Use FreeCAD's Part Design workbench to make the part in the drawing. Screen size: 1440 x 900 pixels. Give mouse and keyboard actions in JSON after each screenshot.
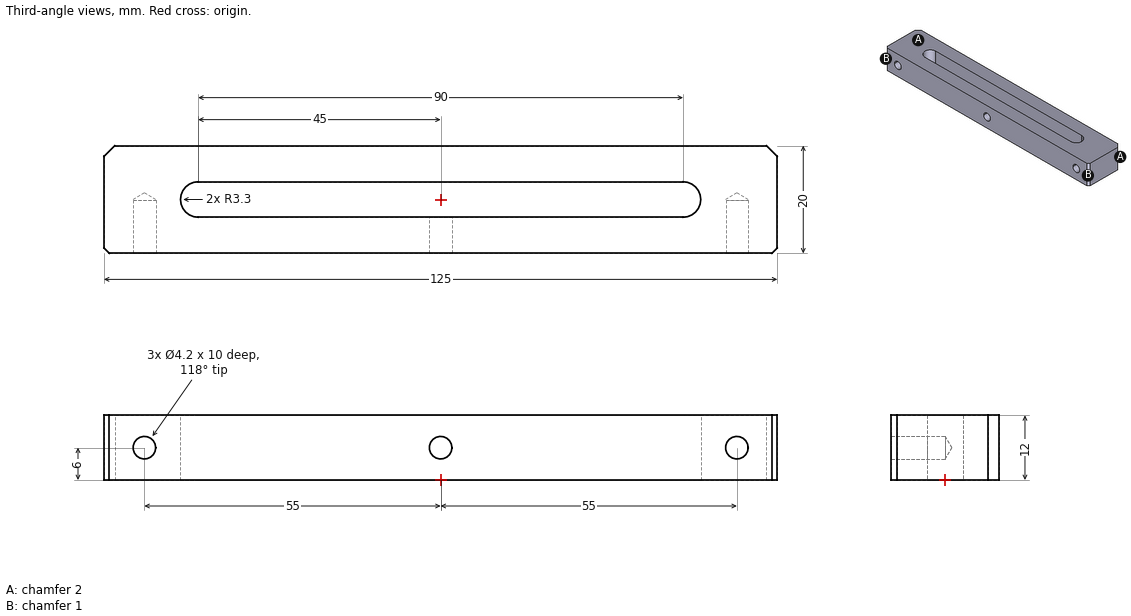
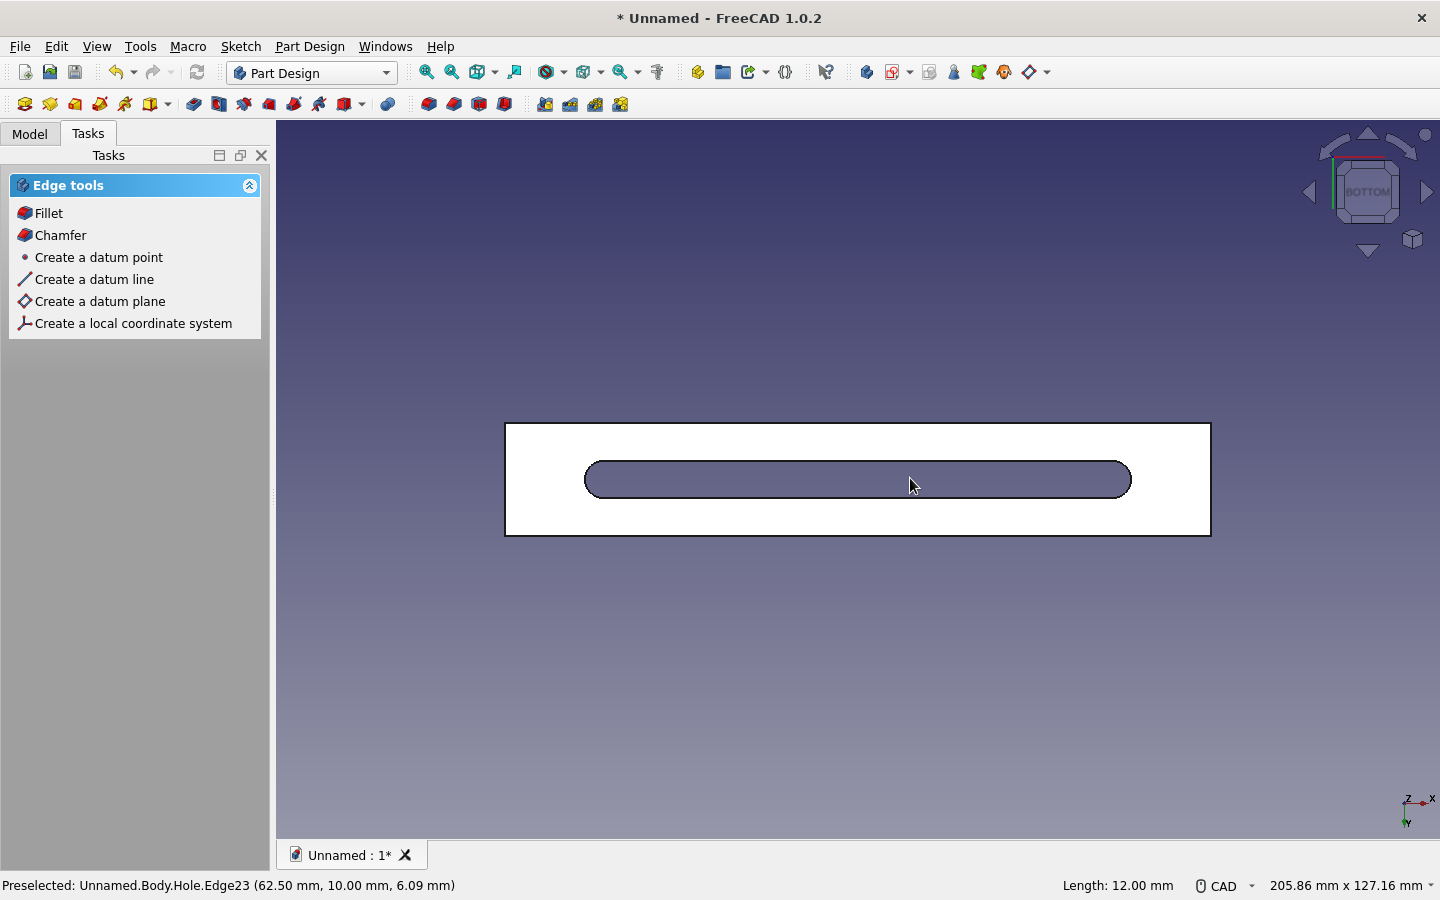
{"action": "key", "text": "4"}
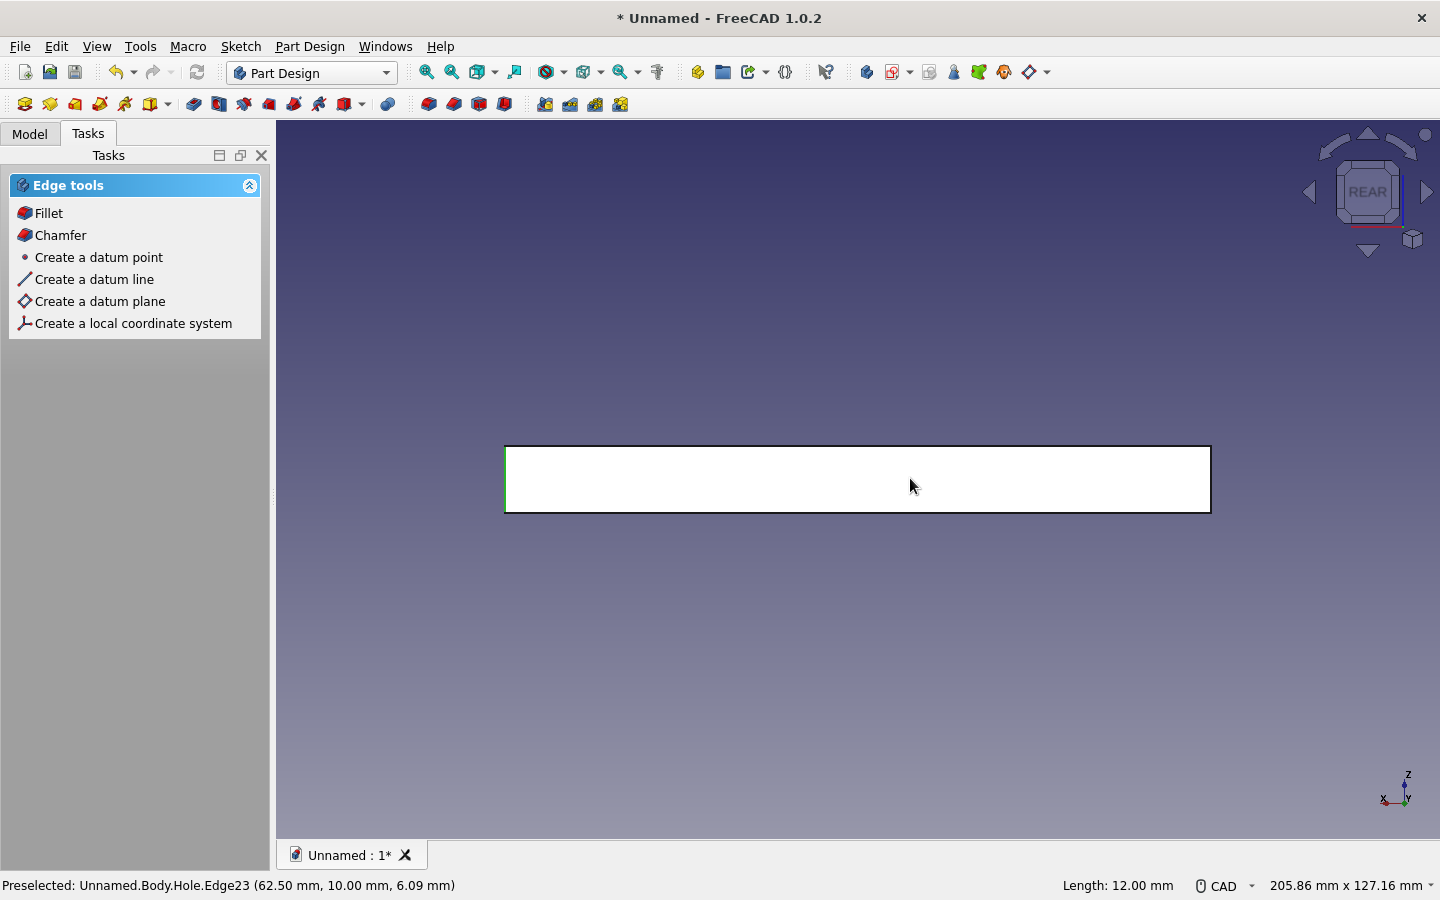
{"action": "left_click", "coordinate": [1211, 479], "text": "ctrl"}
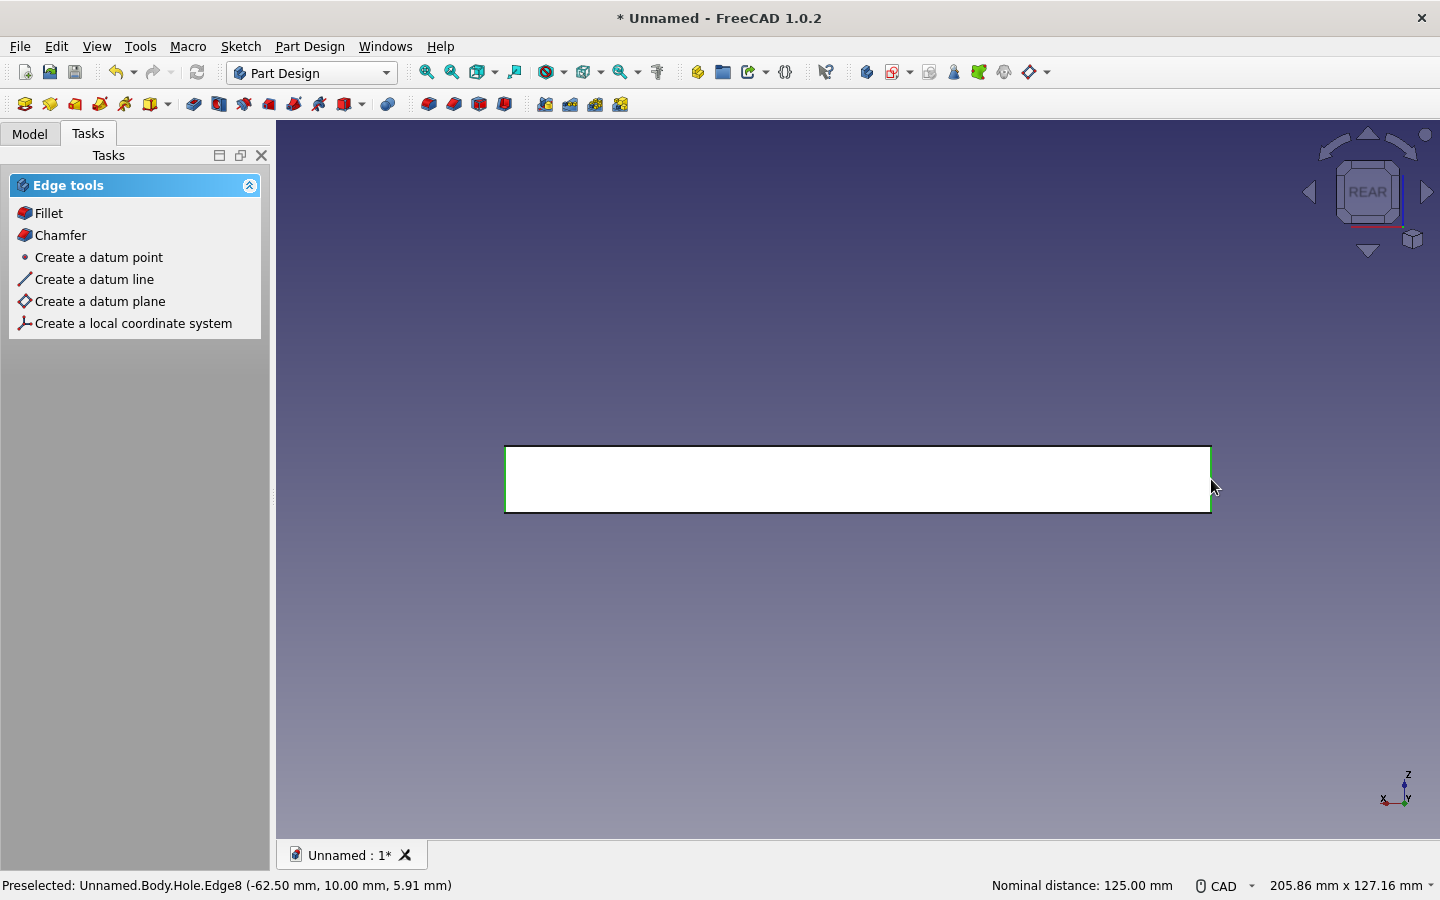
{"action": "left_click", "coordinate": [454, 104]}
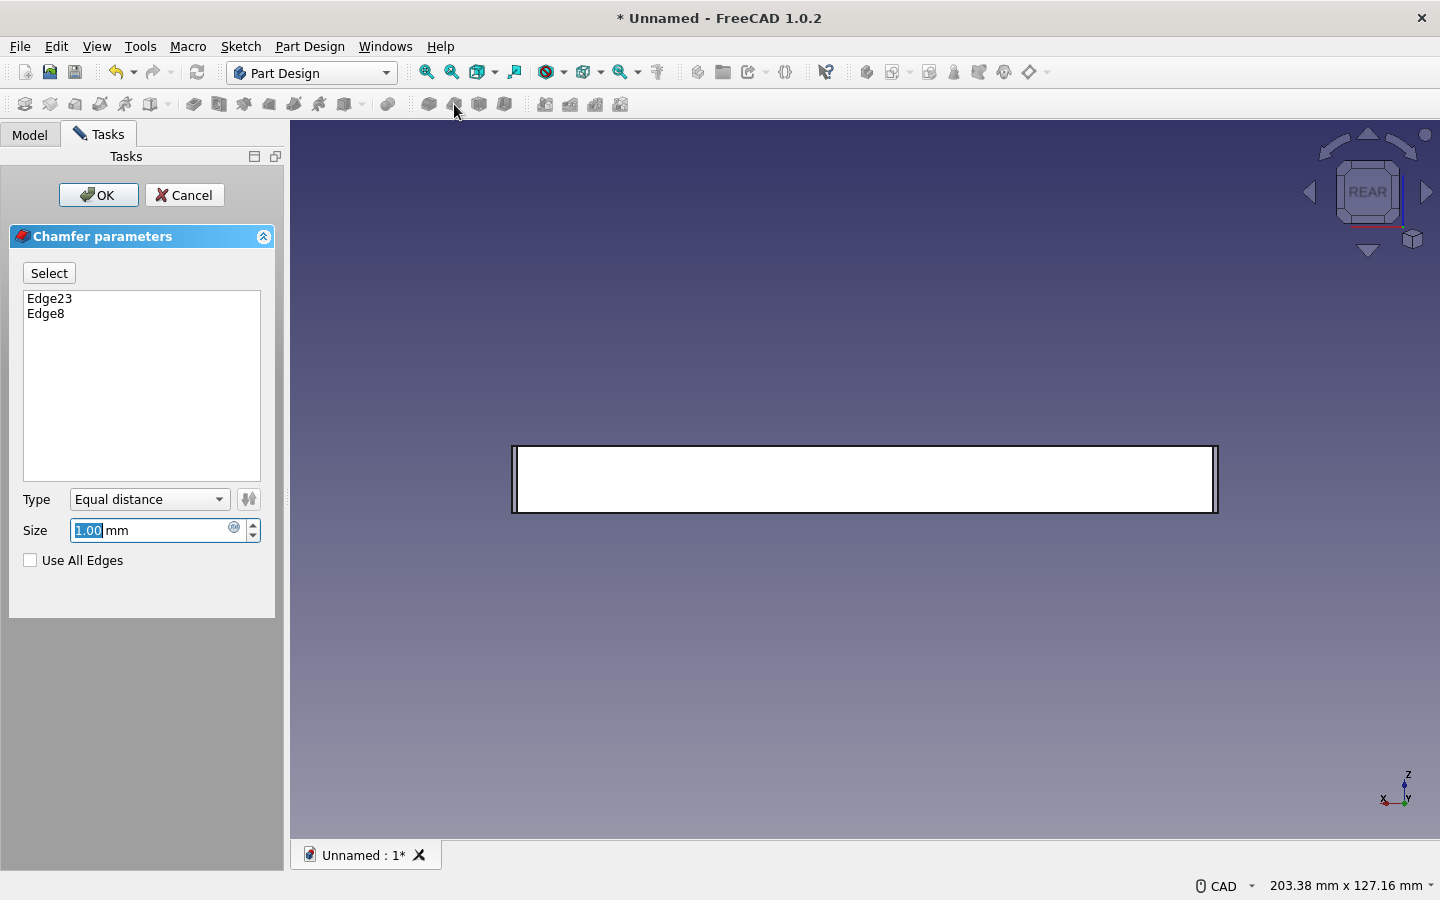
{"action": "type", "text": "2"}
{"action": "key", "text": "Tab"}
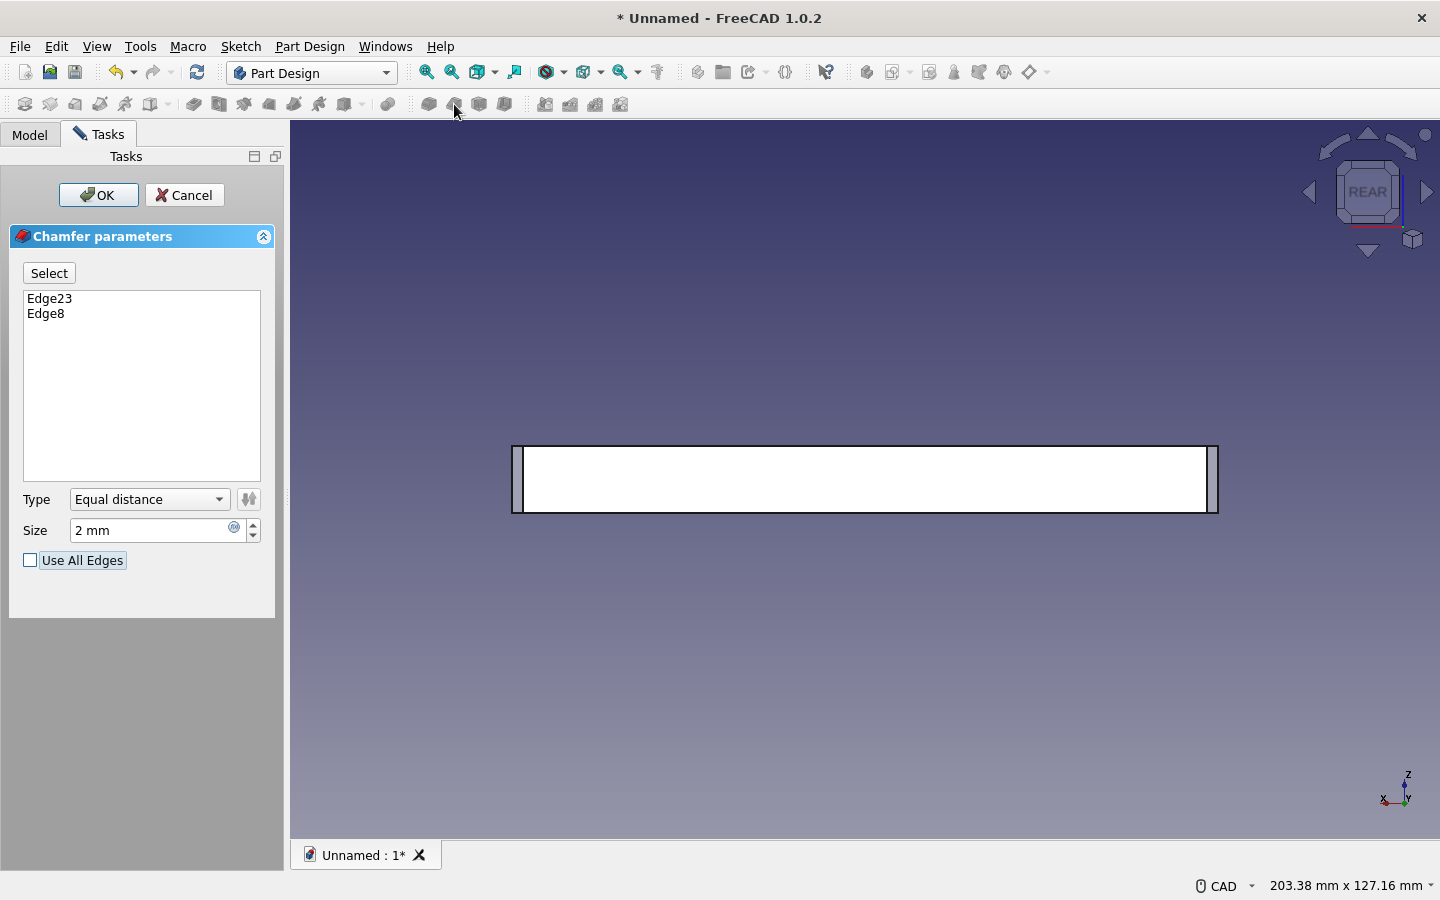
{"action": "left_click", "coordinate": [99, 195]}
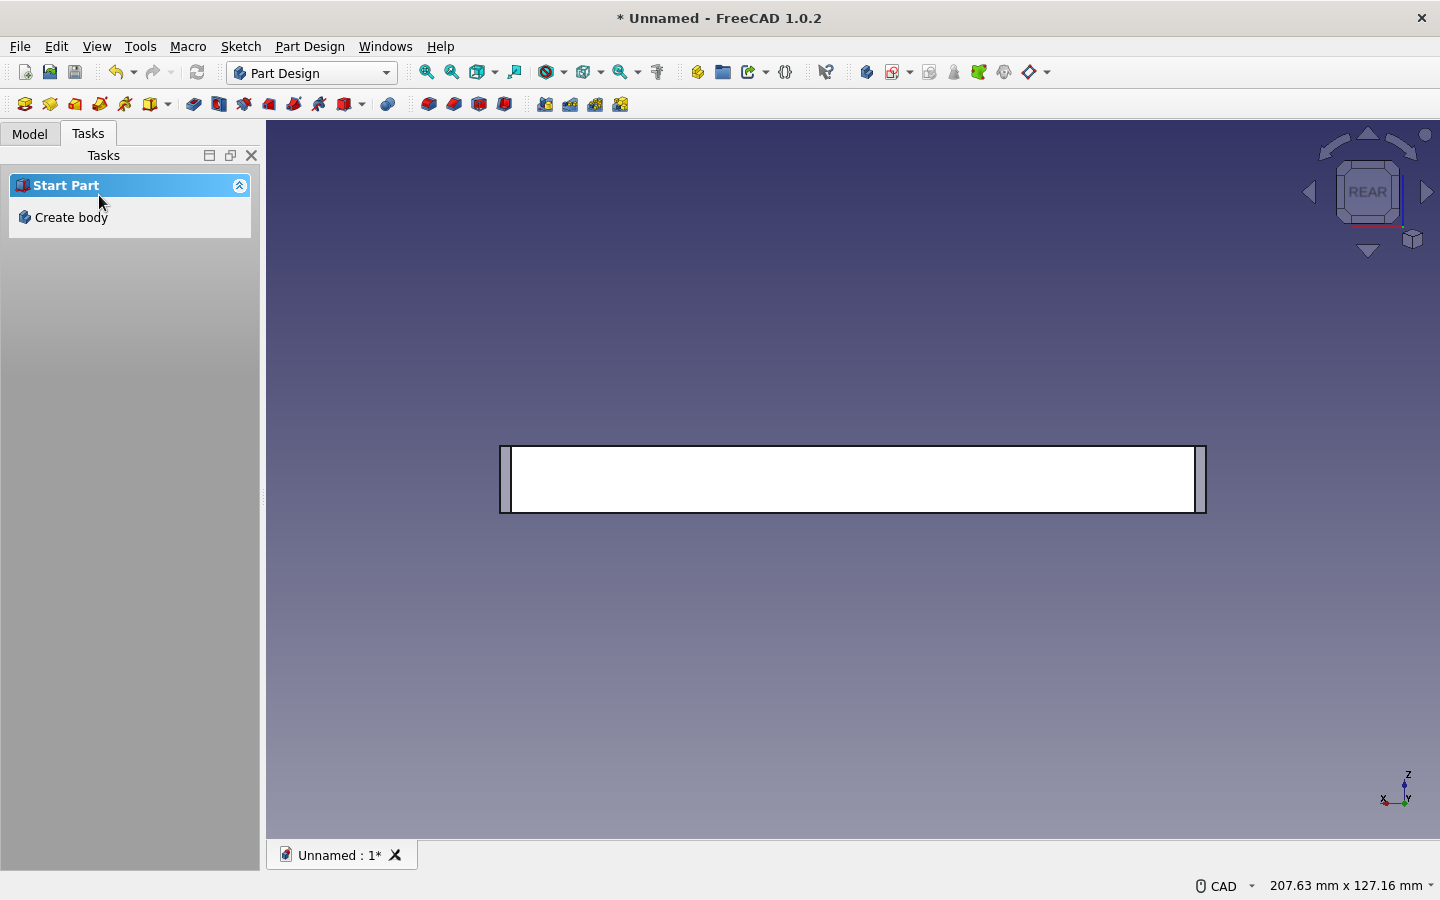
{"action": "key", "text": "0"}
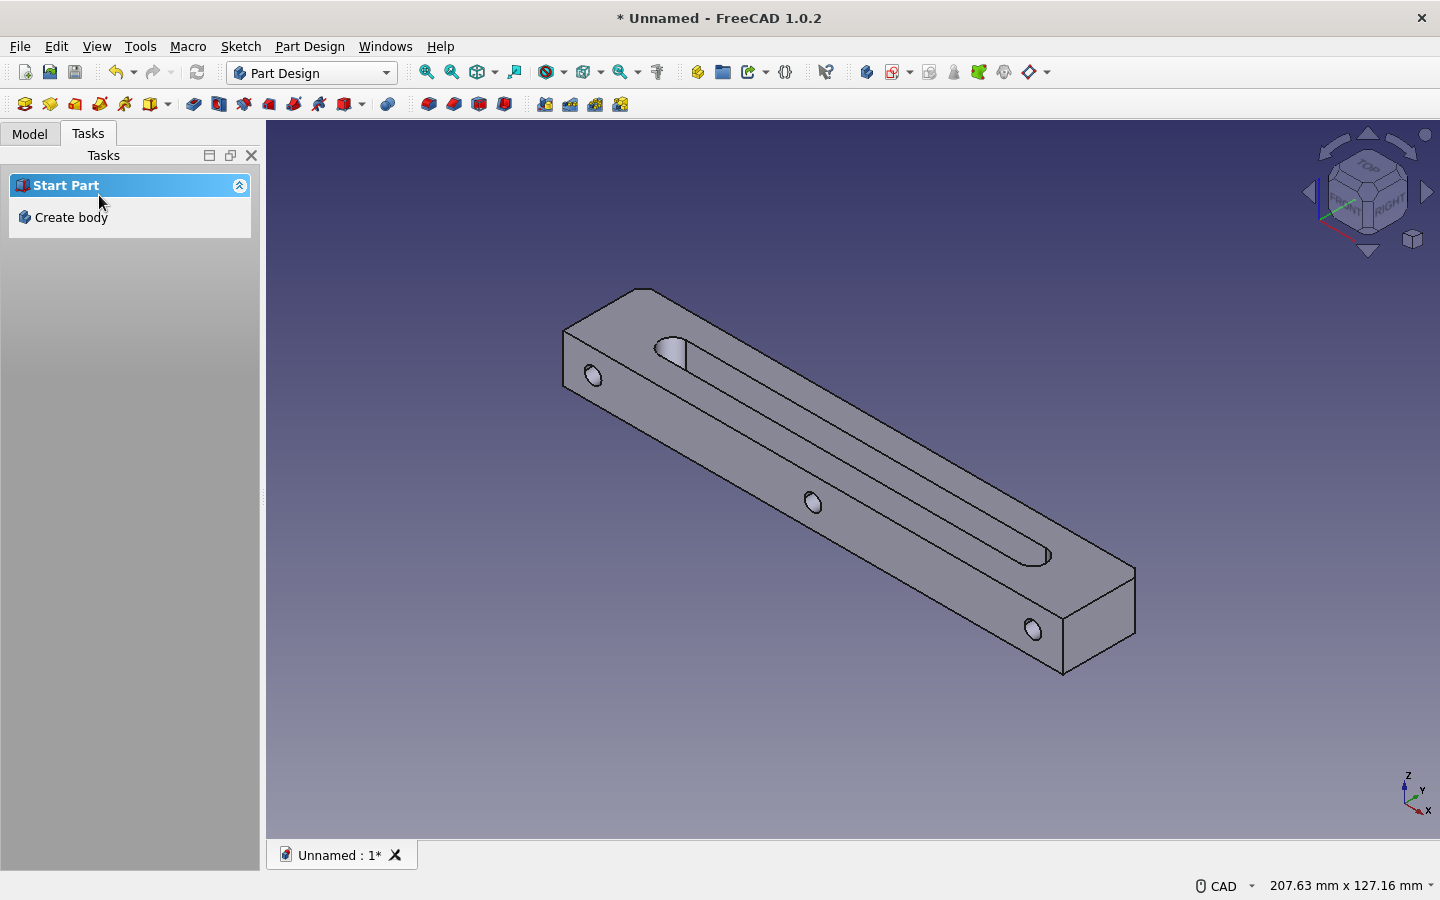
{"action": "left_click", "coordinate": [1063, 646]}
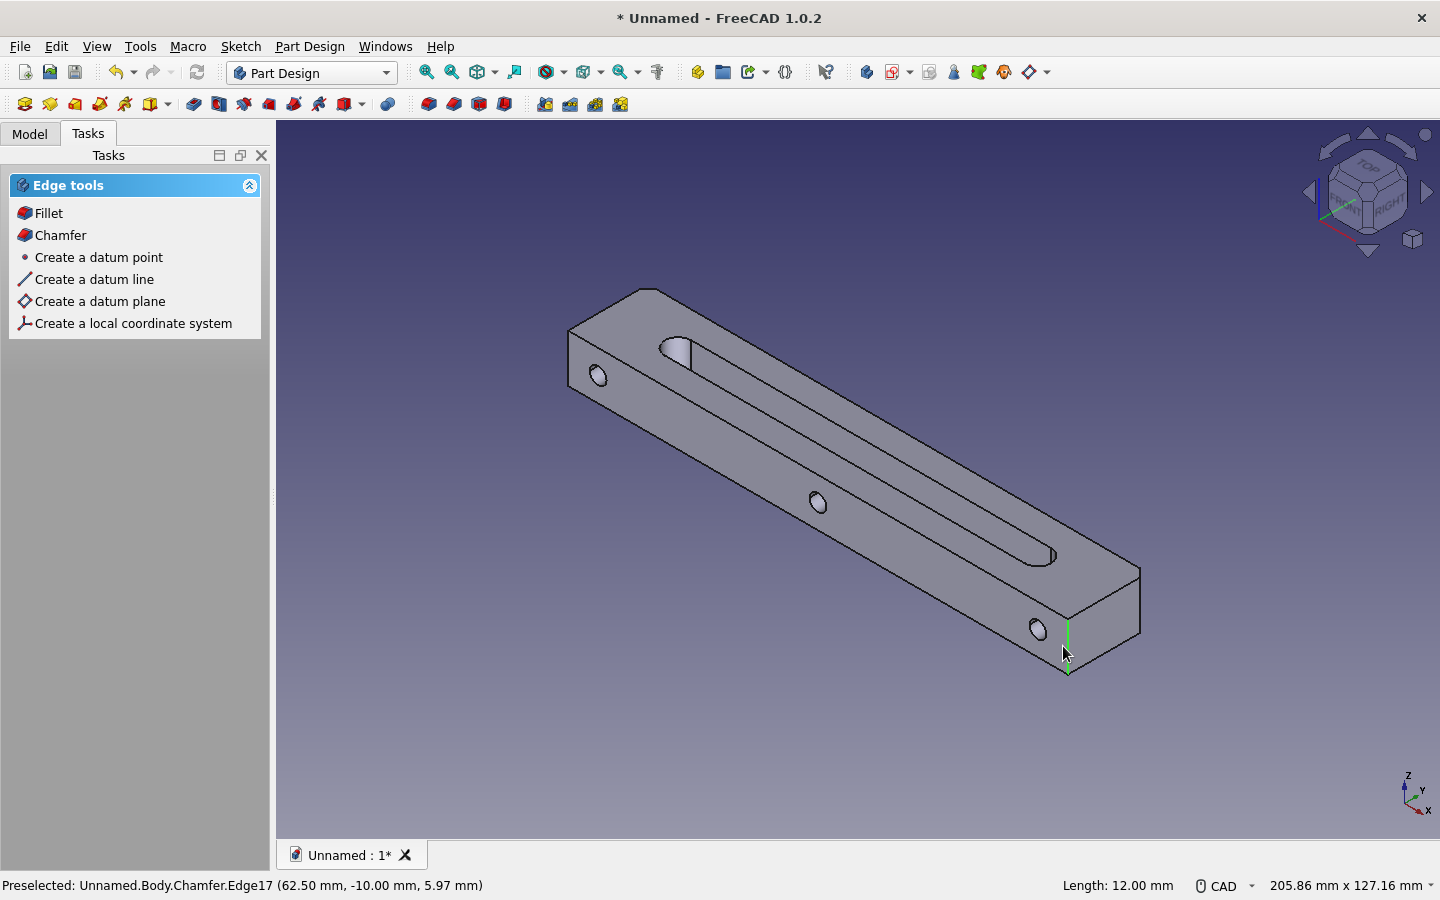
{"action": "key", "text": "2"}